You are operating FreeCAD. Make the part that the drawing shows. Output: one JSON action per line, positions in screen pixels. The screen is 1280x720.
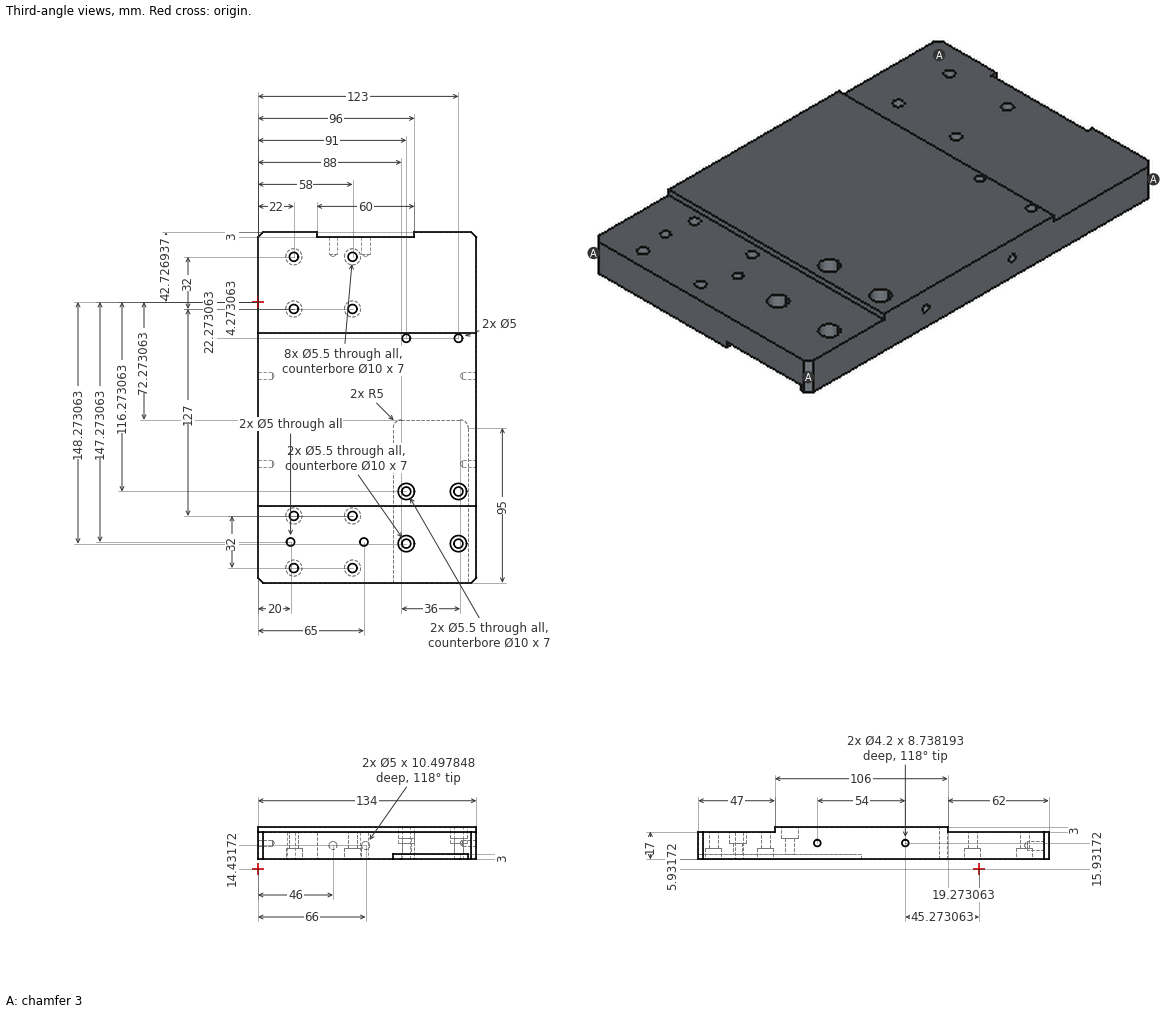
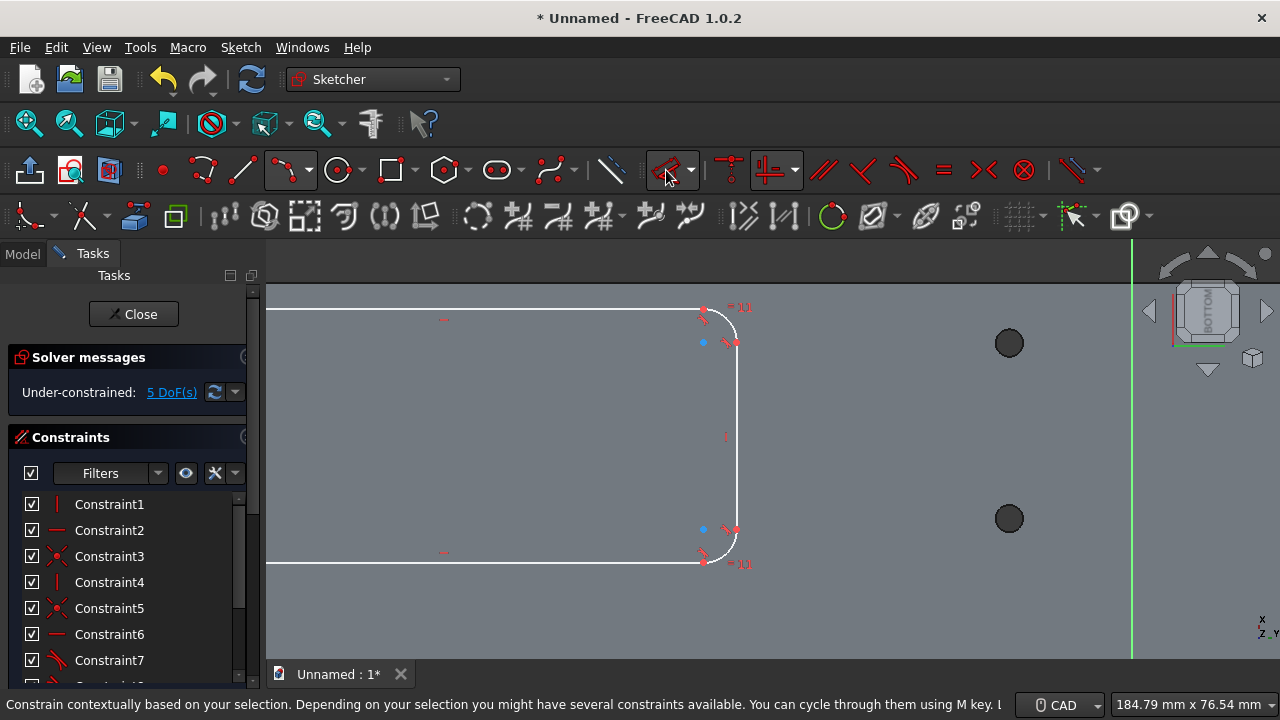
{"action": "scroll", "coordinate": [733, 328], "scroll_direction": "up", "scroll_amount": 2}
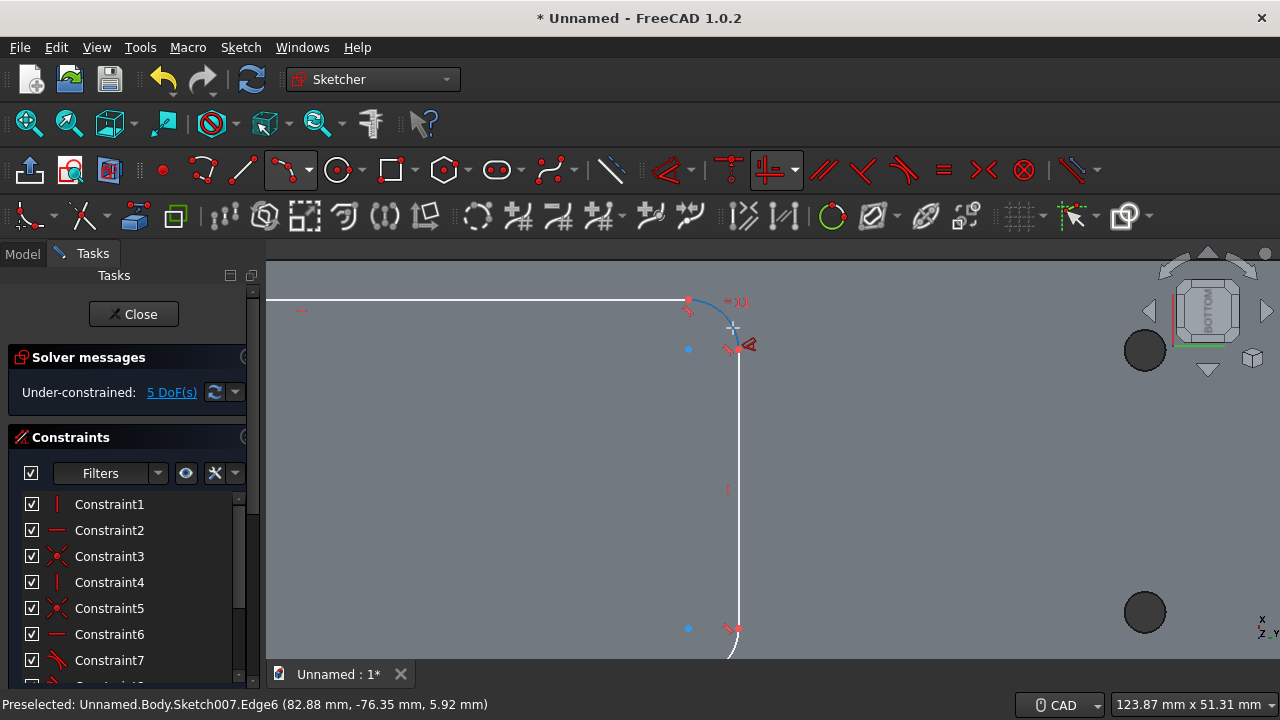
{"action": "left_click", "coordinate": [733, 327]}
{"action": "left_click", "coordinate": [761, 312]}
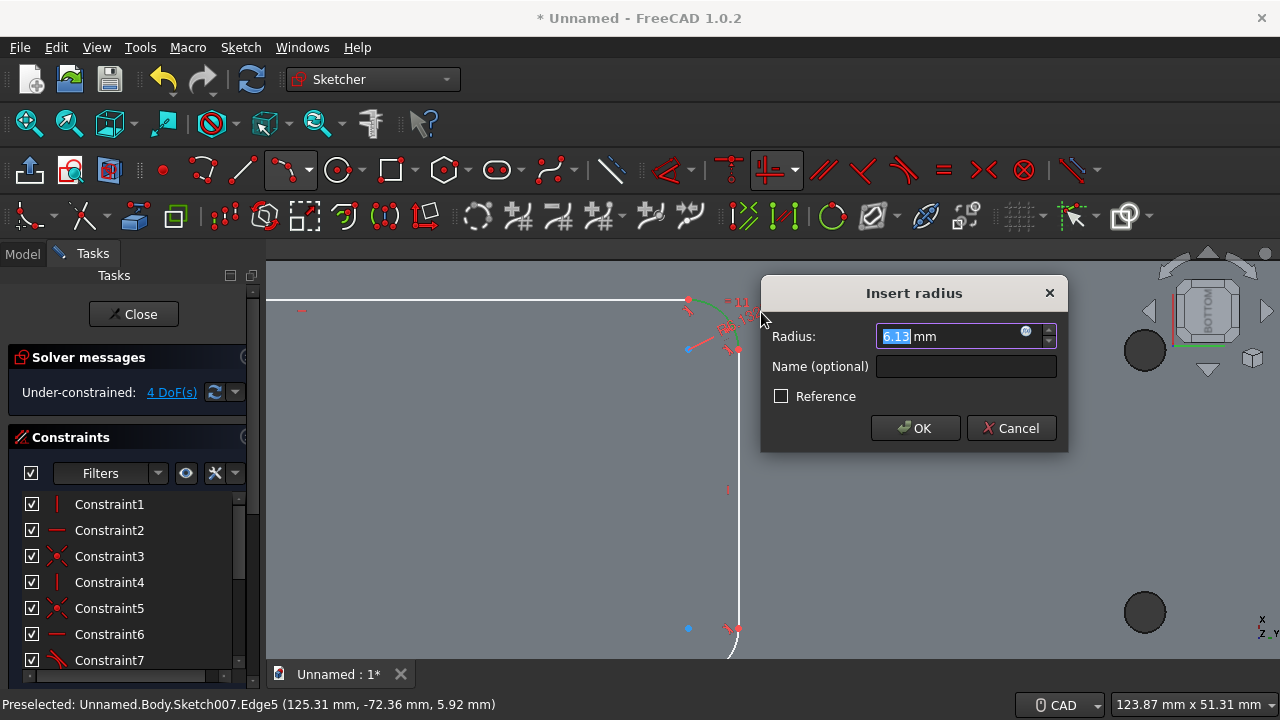
{"action": "type", "text": "5"}
{"action": "key", "text": "Return"}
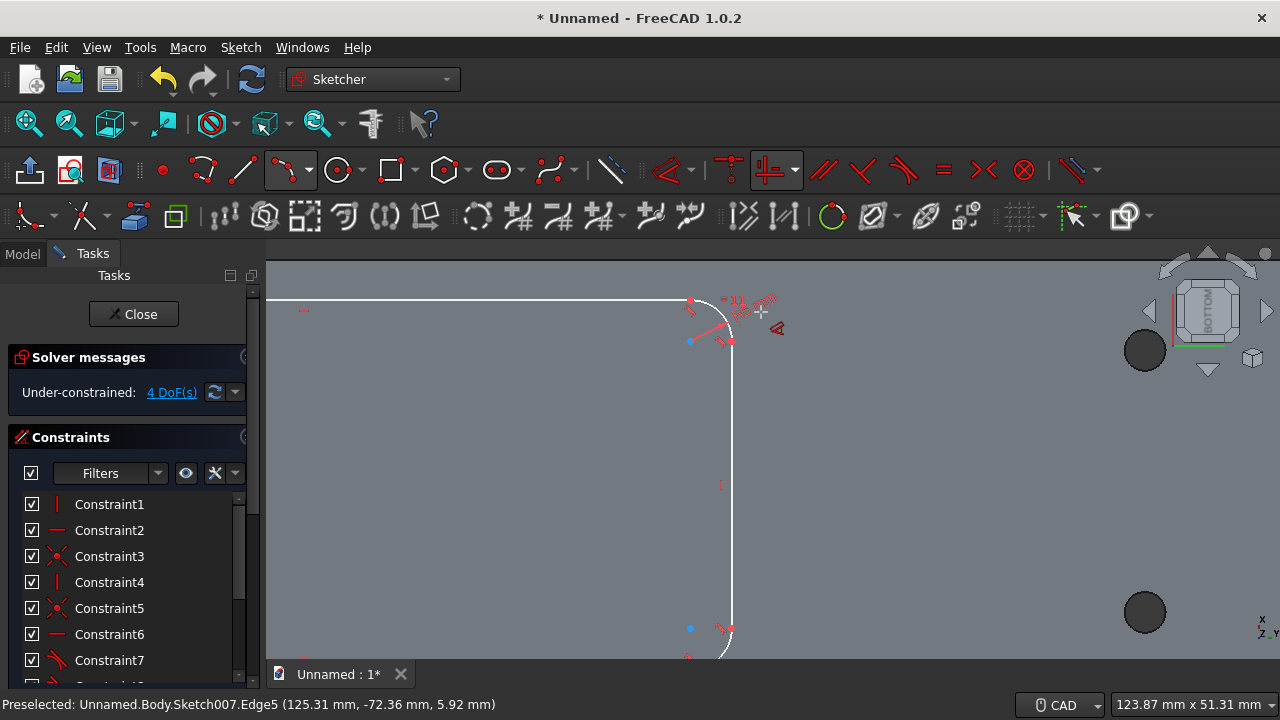
{"action": "scroll", "coordinate": [731, 325], "scroll_direction": "down", "scroll_amount": 7}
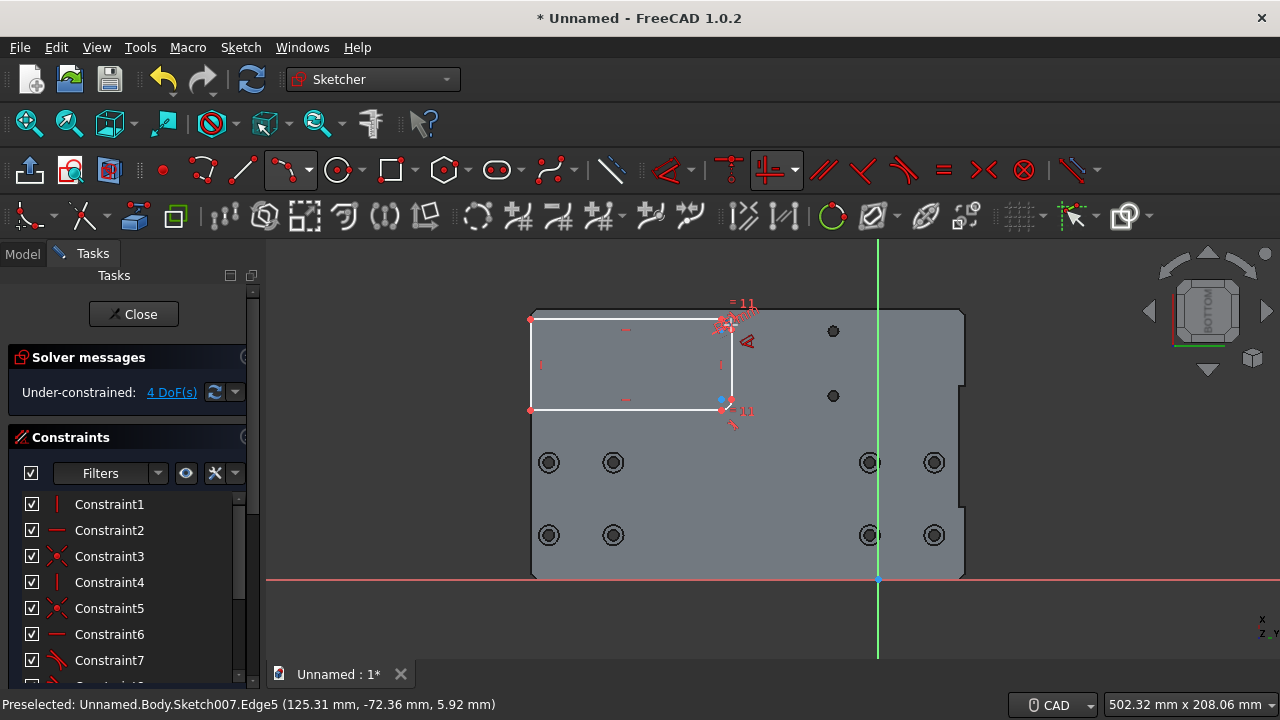
{"action": "left_click", "coordinate": [732, 379]}
{"action": "left_click", "coordinate": [766, 365]}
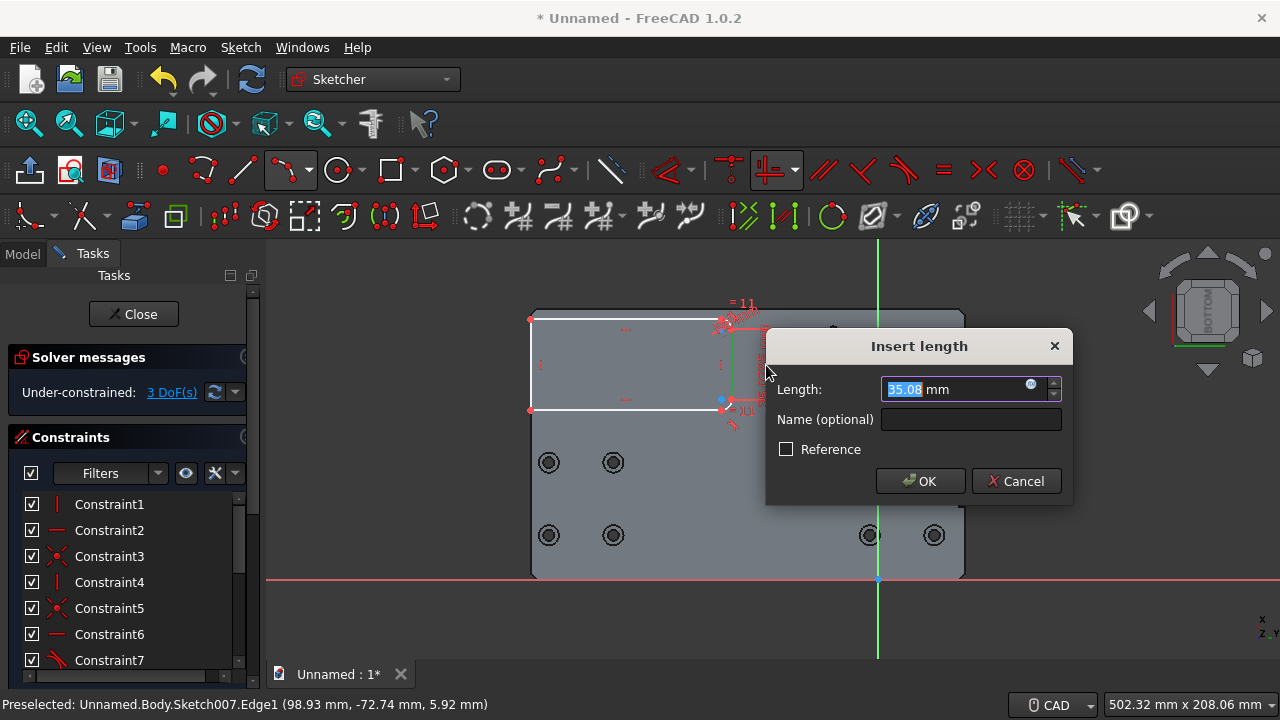
{"action": "type", "text": "36"}
{"action": "key", "text": "Return"}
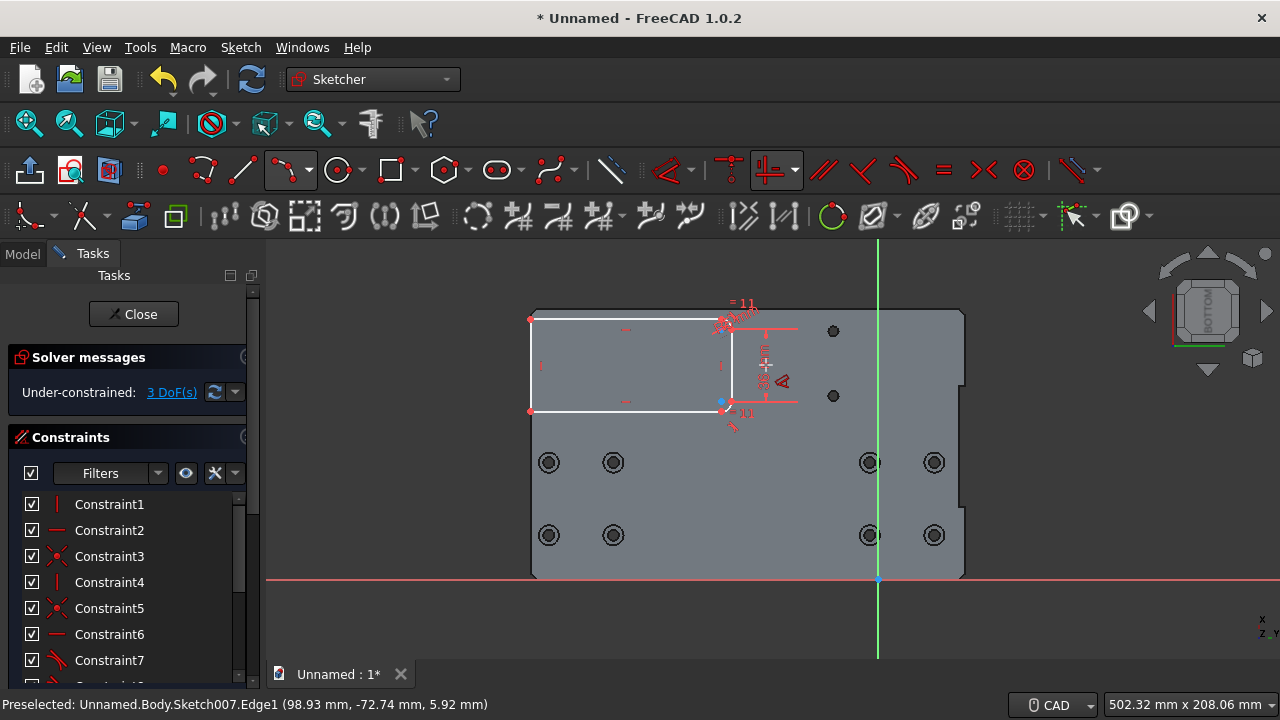
{"action": "left_click", "coordinate": [664, 319]}
{"action": "left_click", "coordinate": [626, 285]}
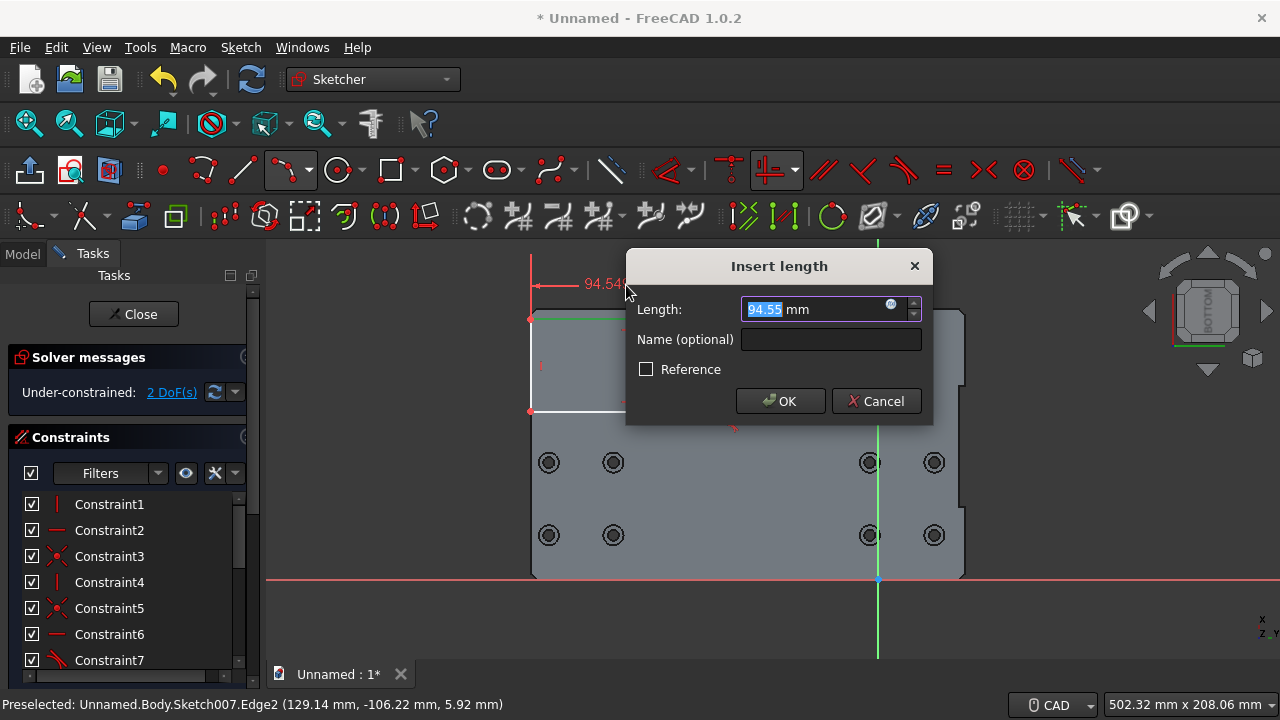
{"action": "type", "text": "95"}
{"action": "key", "text": "Return"}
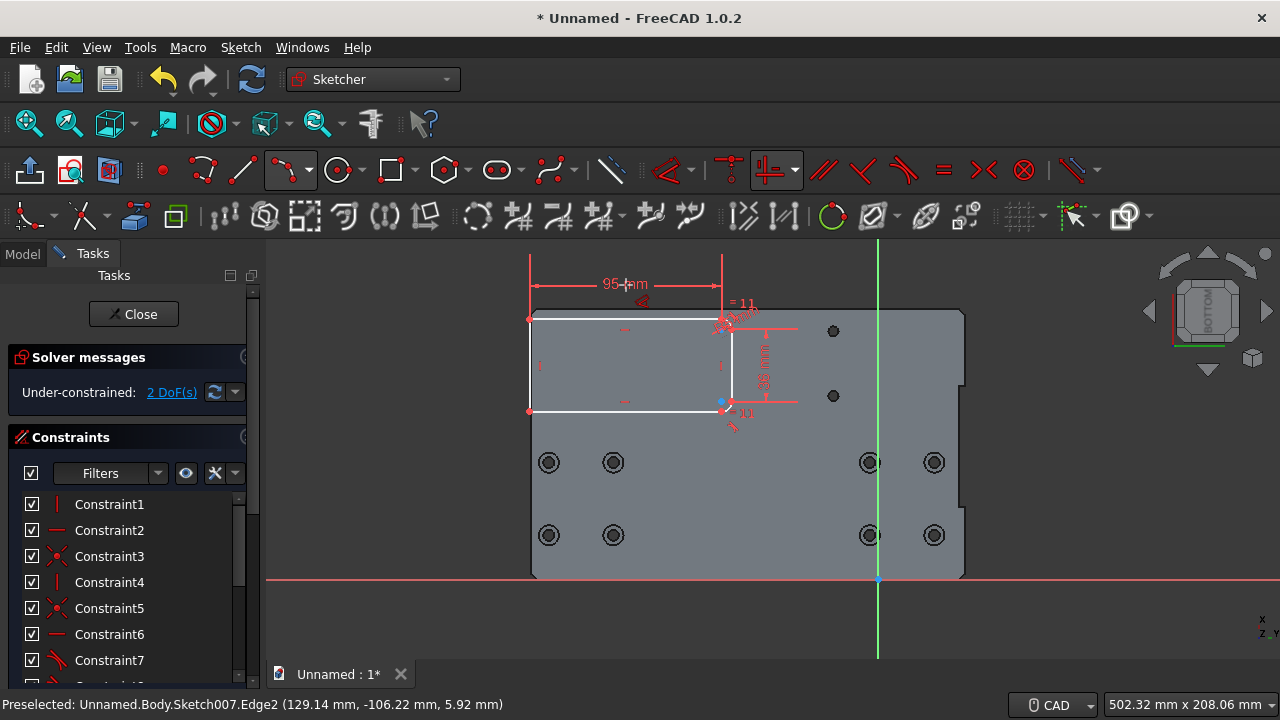
{"action": "left_click", "coordinate": [732, 402]}
{"action": "left_click", "coordinate": [912, 491]}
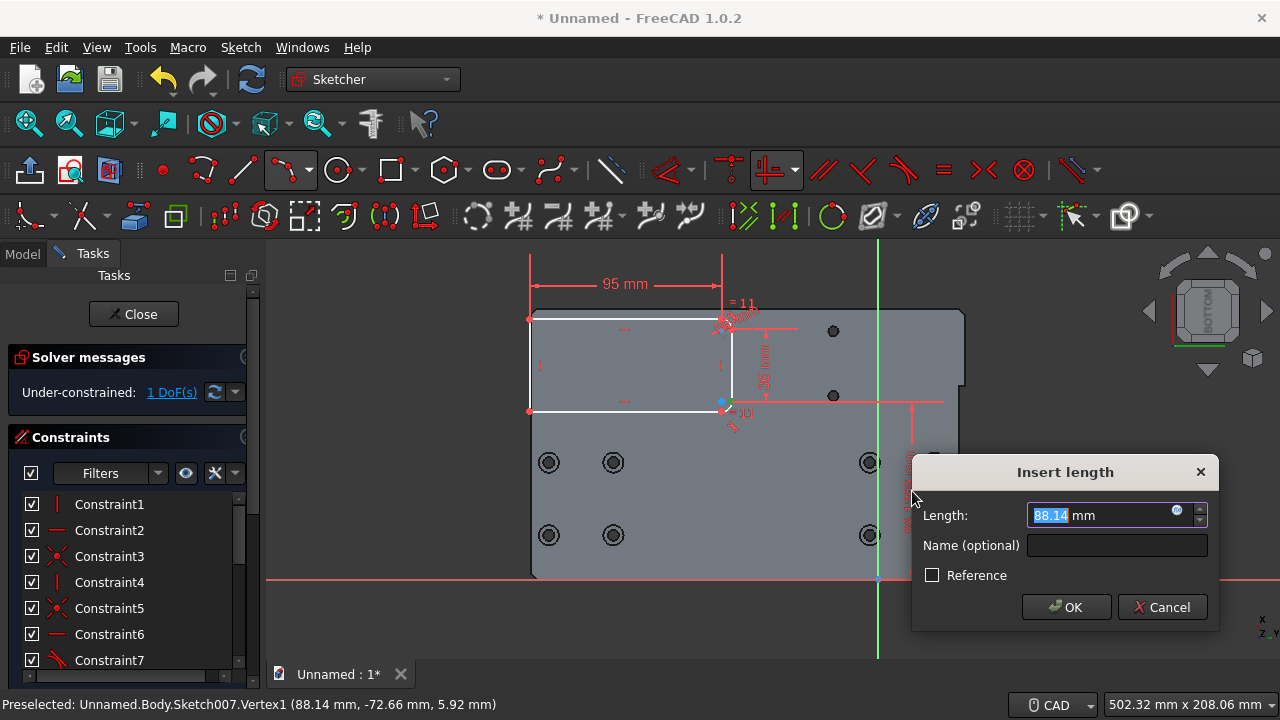
{"action": "type", "text": "88"}
{"action": "key", "text": "Return"}